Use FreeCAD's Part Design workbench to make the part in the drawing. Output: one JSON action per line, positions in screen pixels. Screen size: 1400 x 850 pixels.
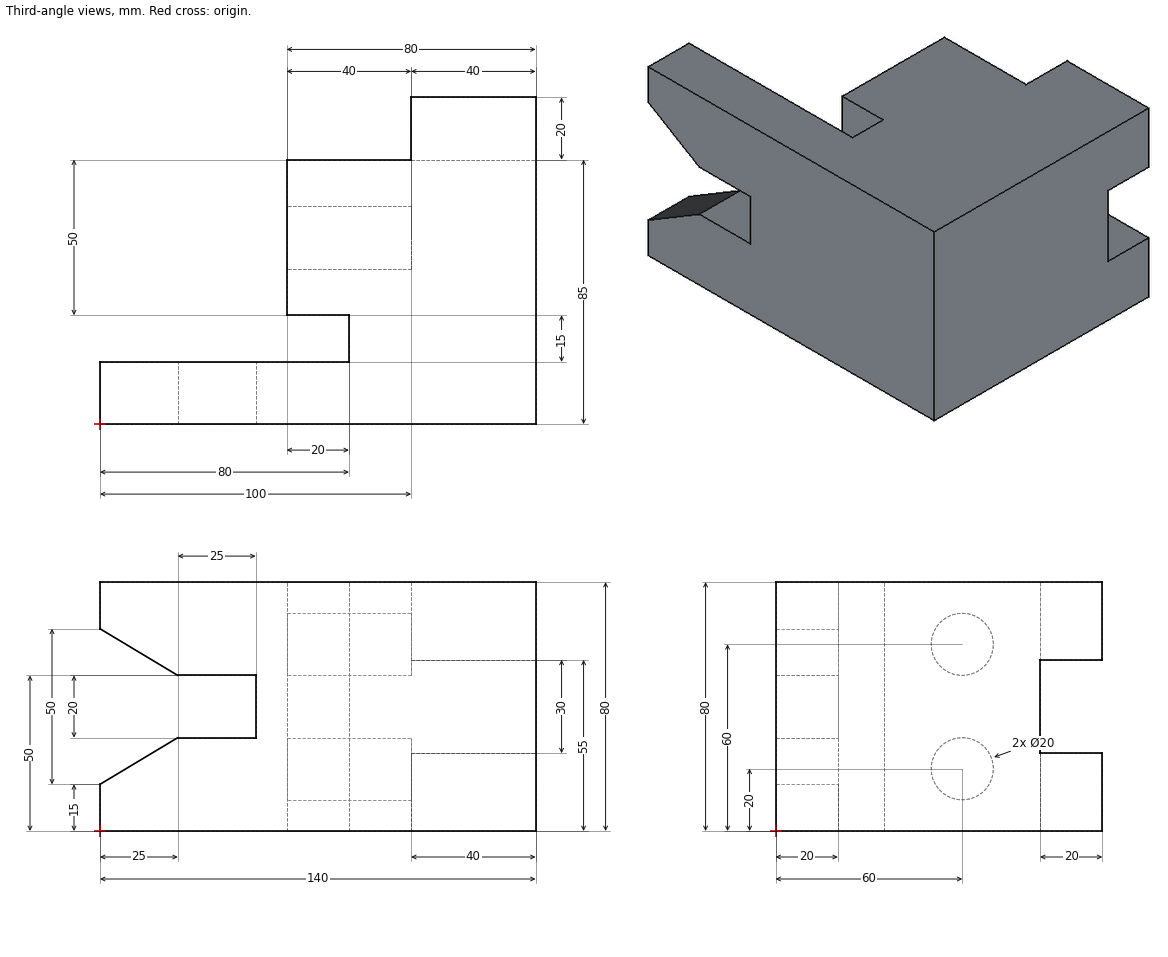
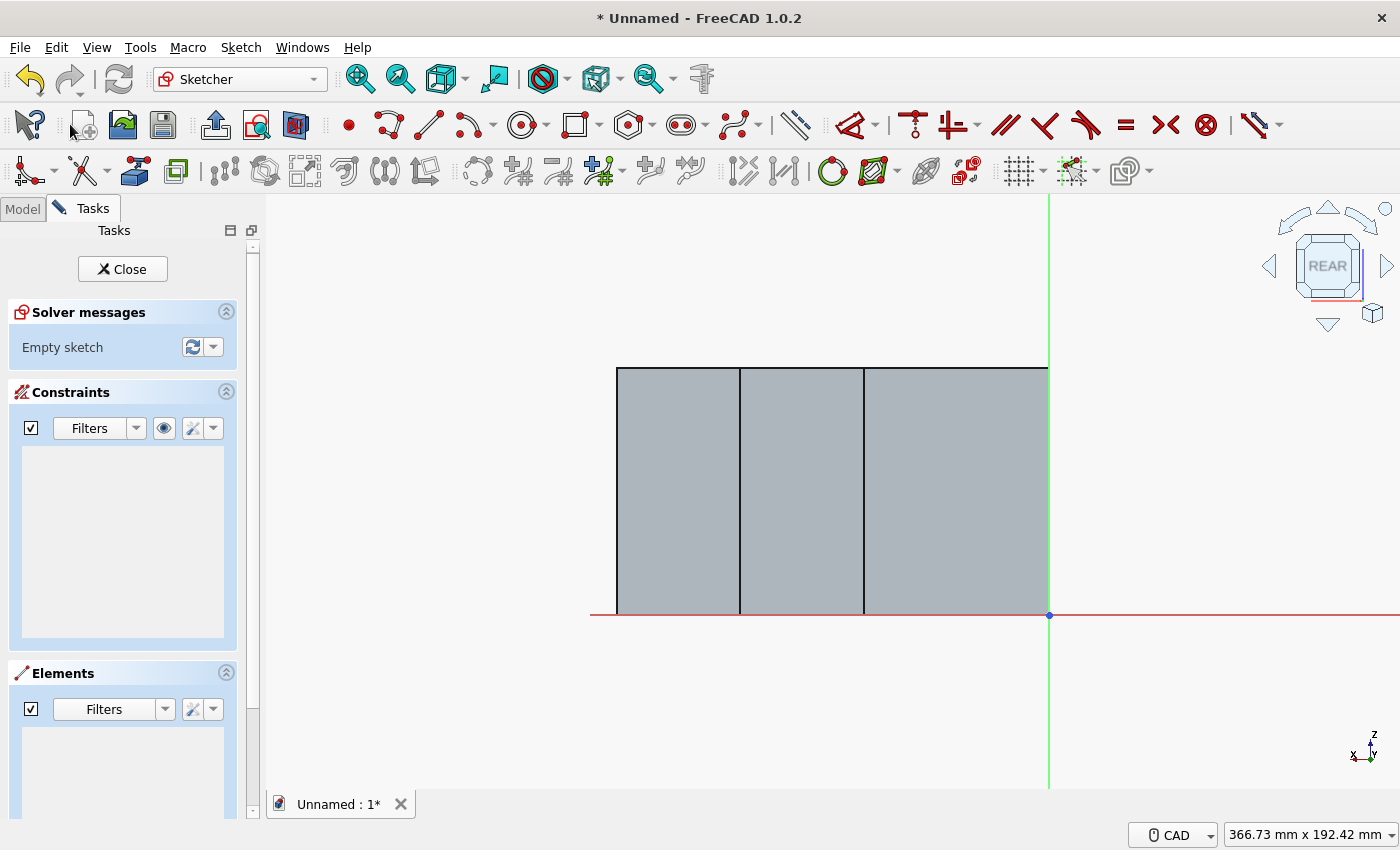
{"action": "scroll", "coordinate": [650, 492], "scroll_direction": "up", "scroll_amount": 7}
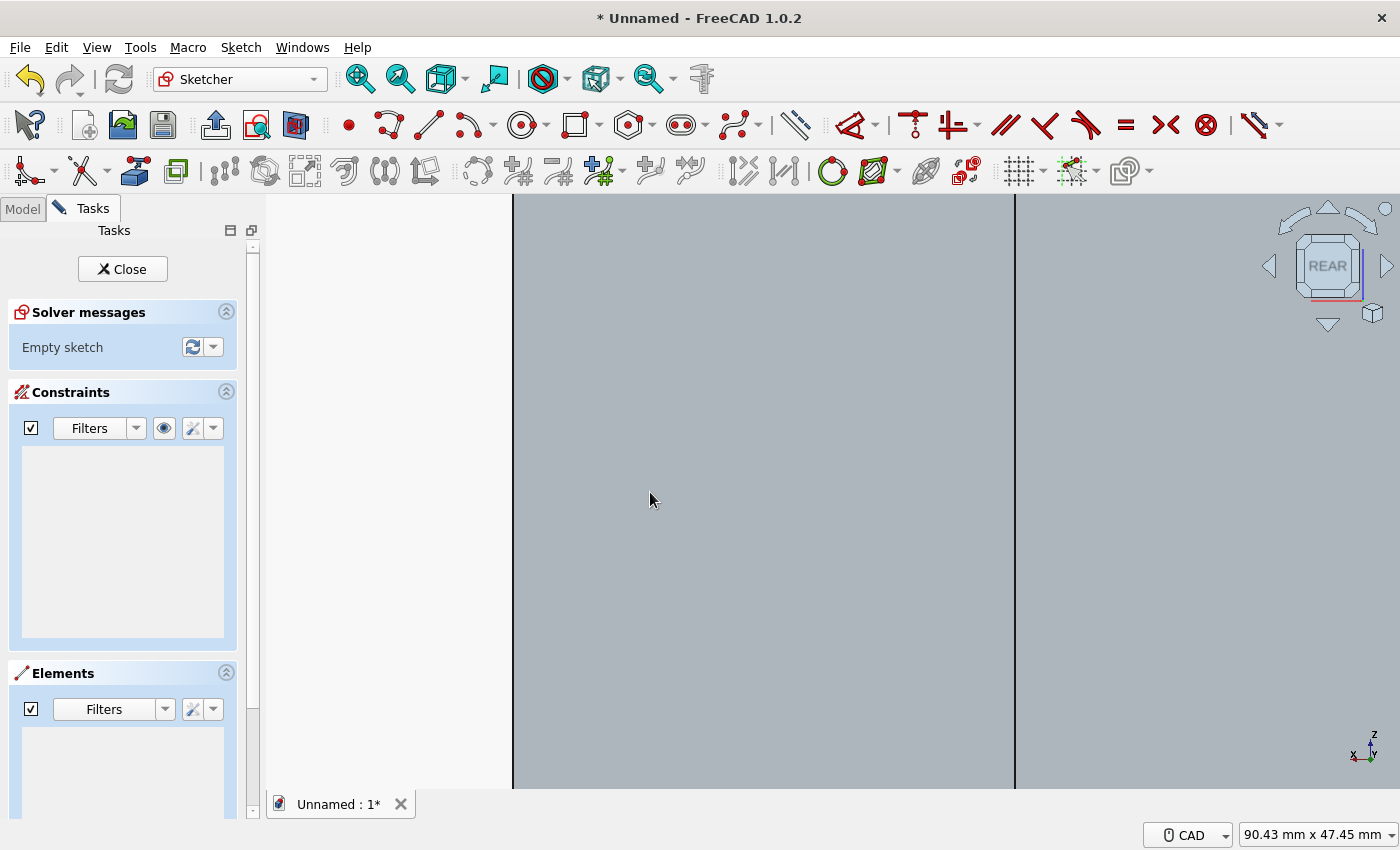
{"action": "key", "text": "g r"}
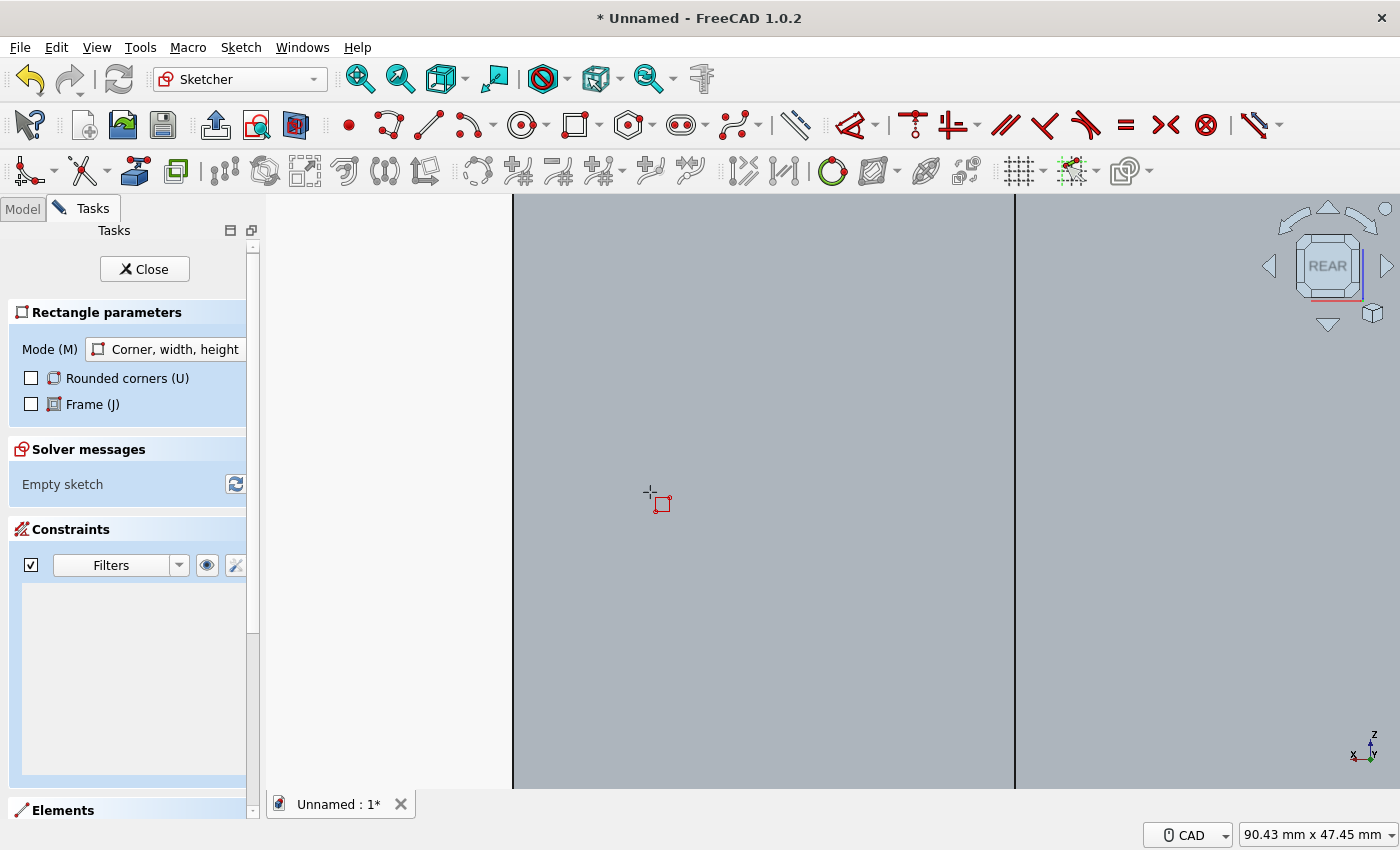
{"action": "left_click", "coordinate": [513, 300]}
{"action": "mouse_move", "coordinate": [1015, 677]}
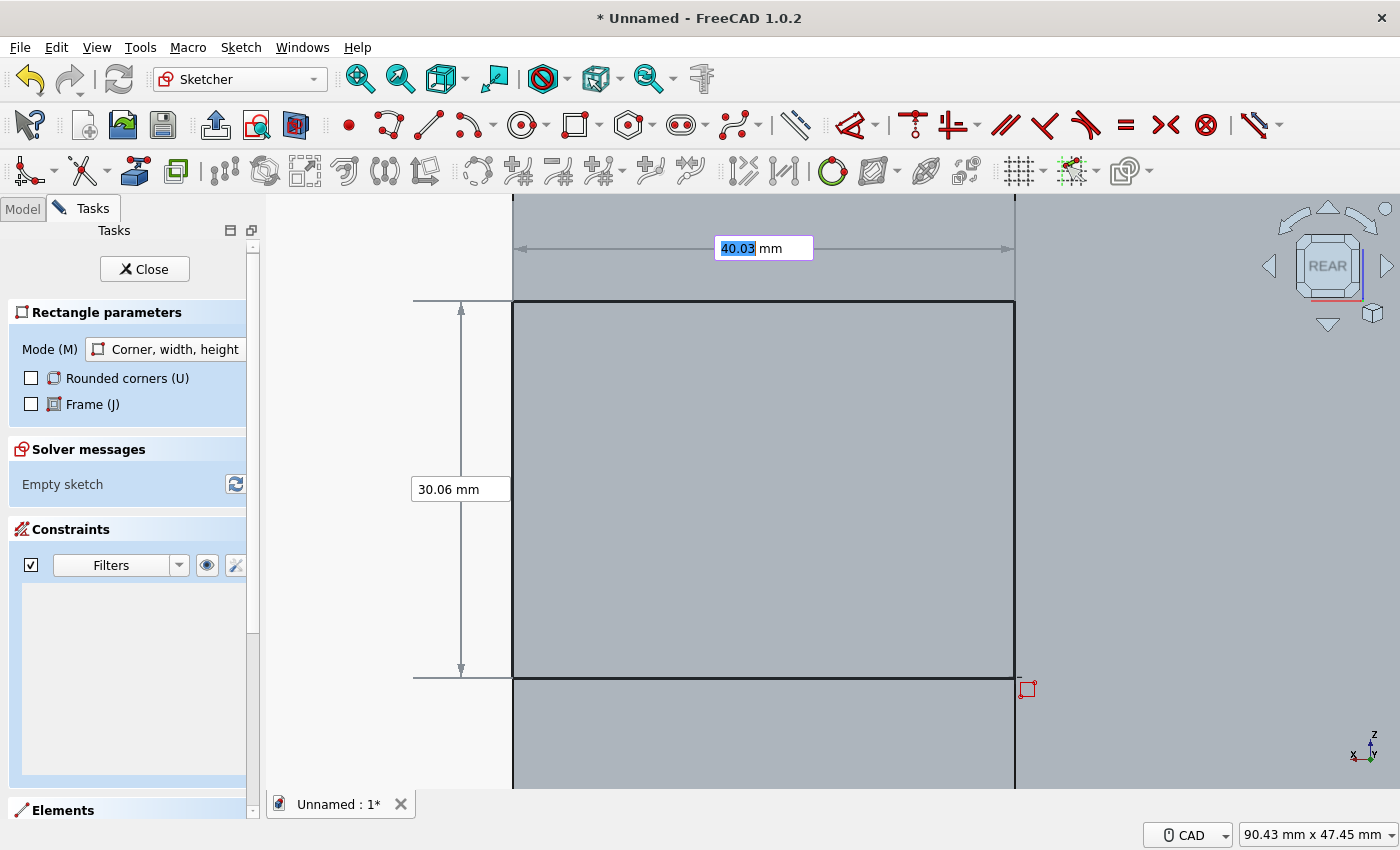
{"action": "type", "text": "40"}
{"action": "key", "text": "Tab"}
{"action": "type", "text": "30"}
{"action": "key", "text": "Return"}
{"action": "key", "text": "Escape"}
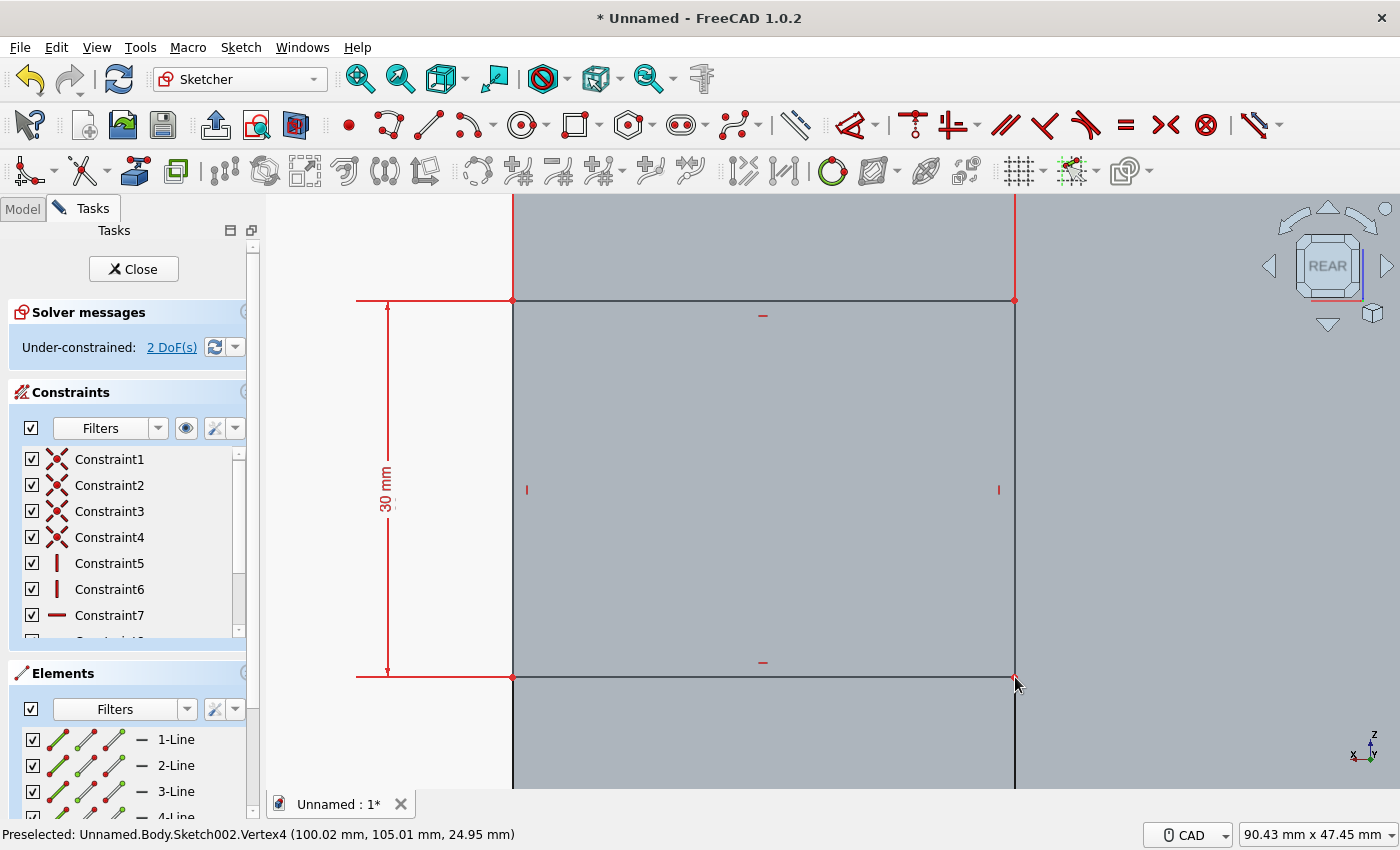
{"action": "key", "text": "d"}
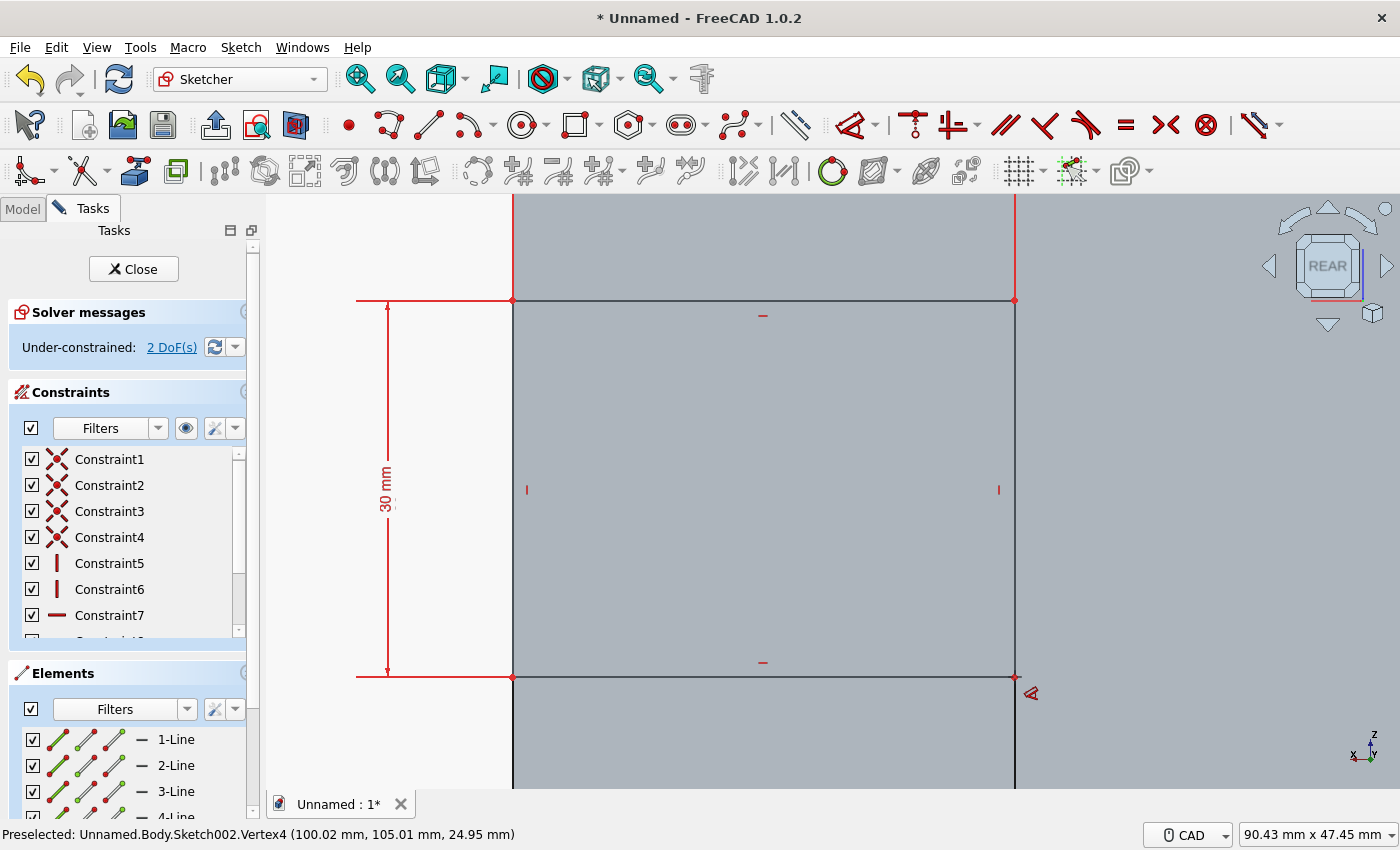
{"action": "left_click", "coordinate": [513, 301]}
{"action": "left_click", "coordinate": [479, 531]}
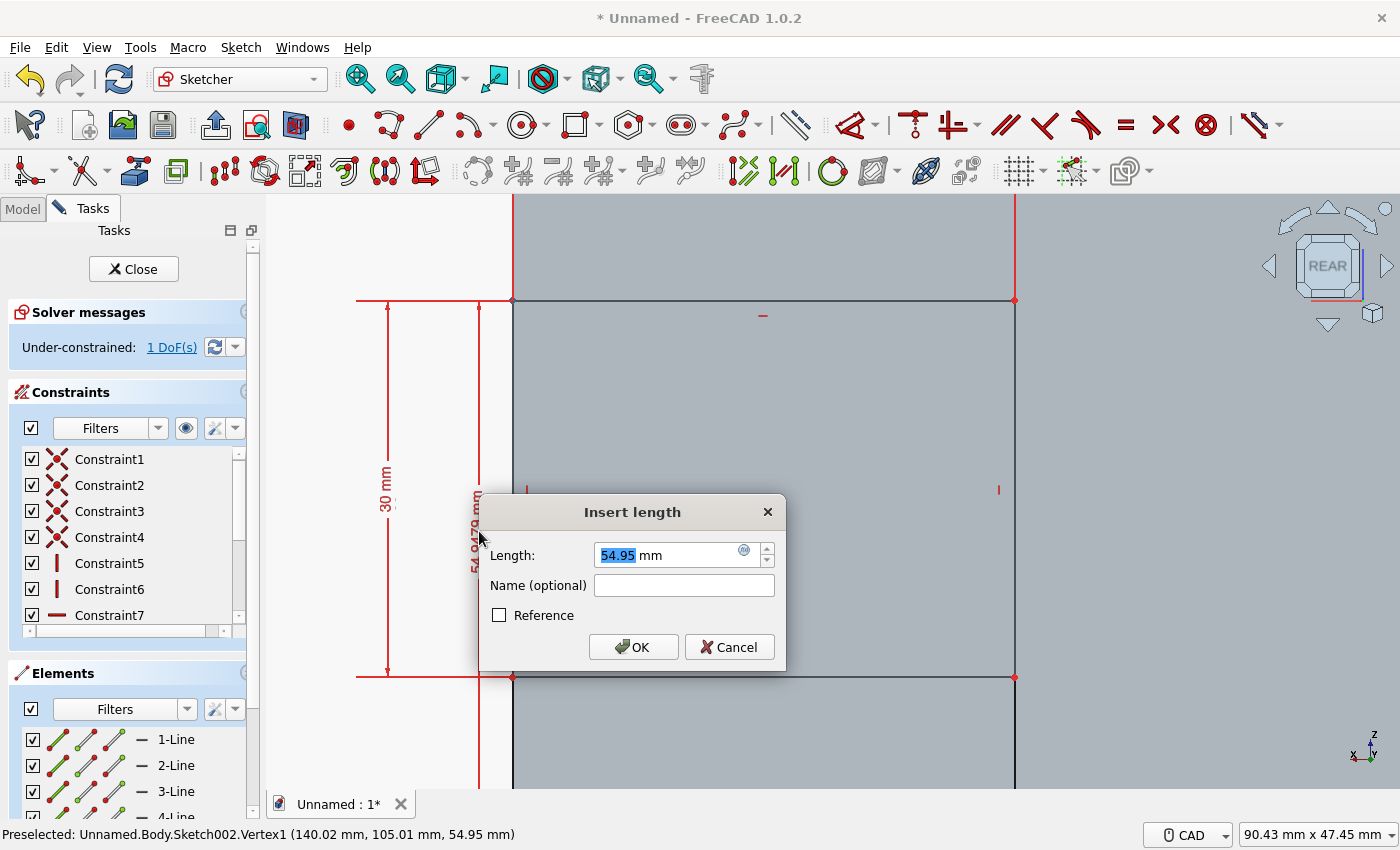
{"action": "type", "text": "55"}
{"action": "key", "text": "Return"}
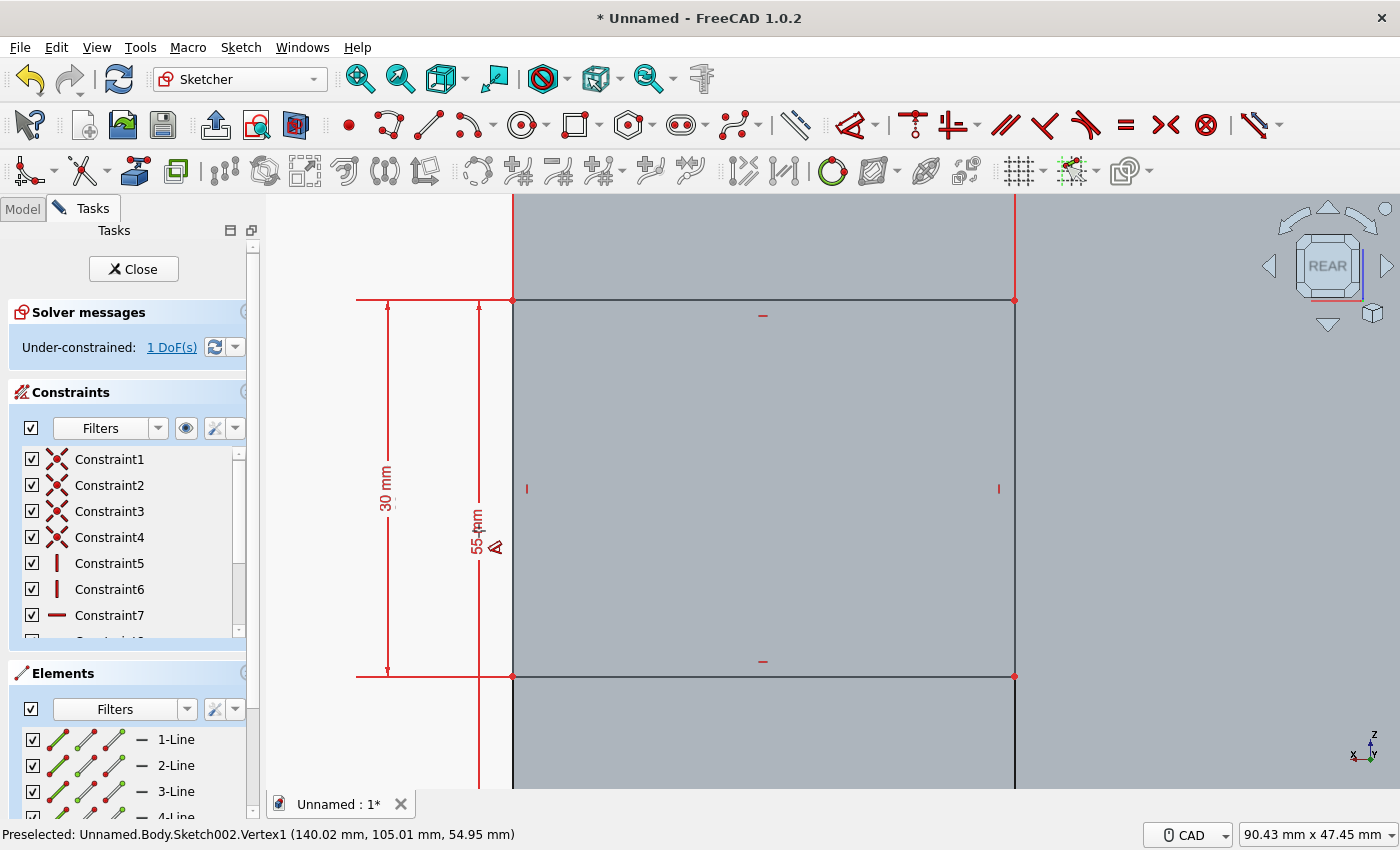
{"action": "left_click", "coordinate": [513, 300]}
{"action": "left_click", "coordinate": [874, 266]}